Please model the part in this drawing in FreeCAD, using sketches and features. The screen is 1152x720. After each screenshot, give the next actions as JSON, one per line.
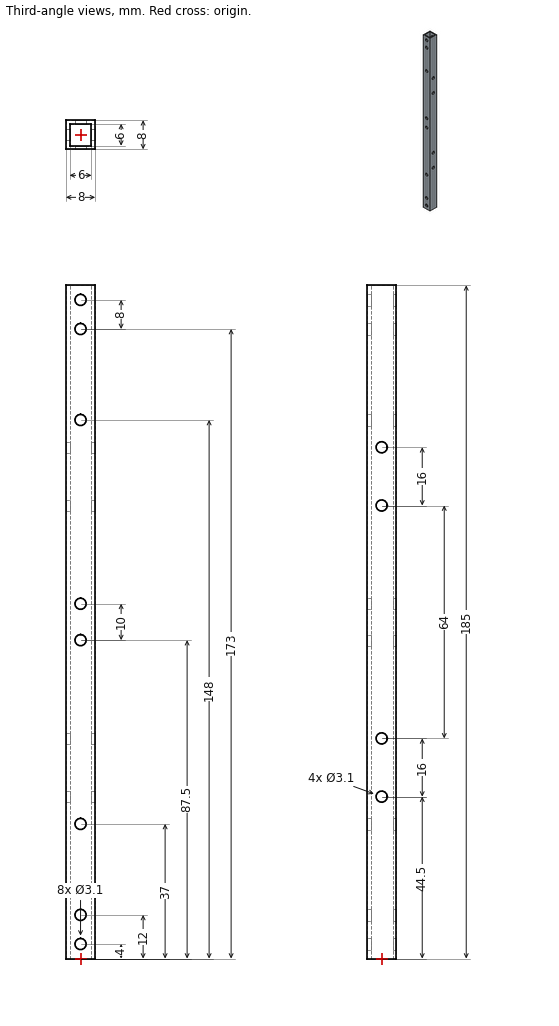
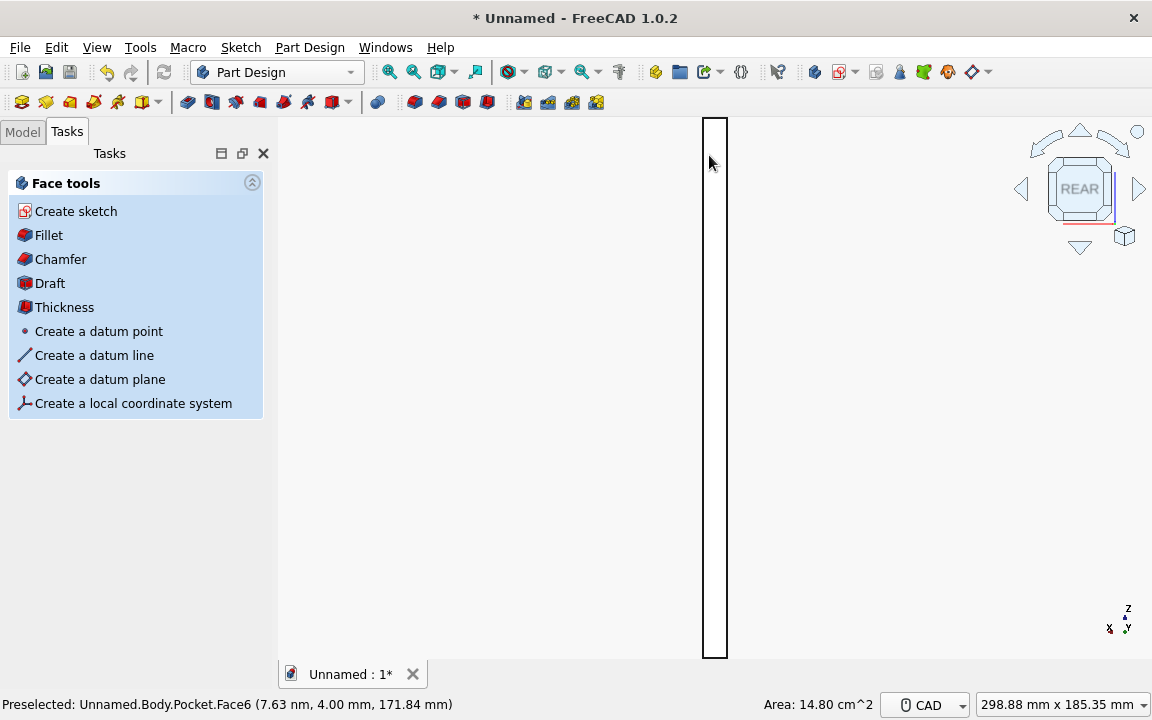
{"action": "left_click", "coordinate": [840, 72]}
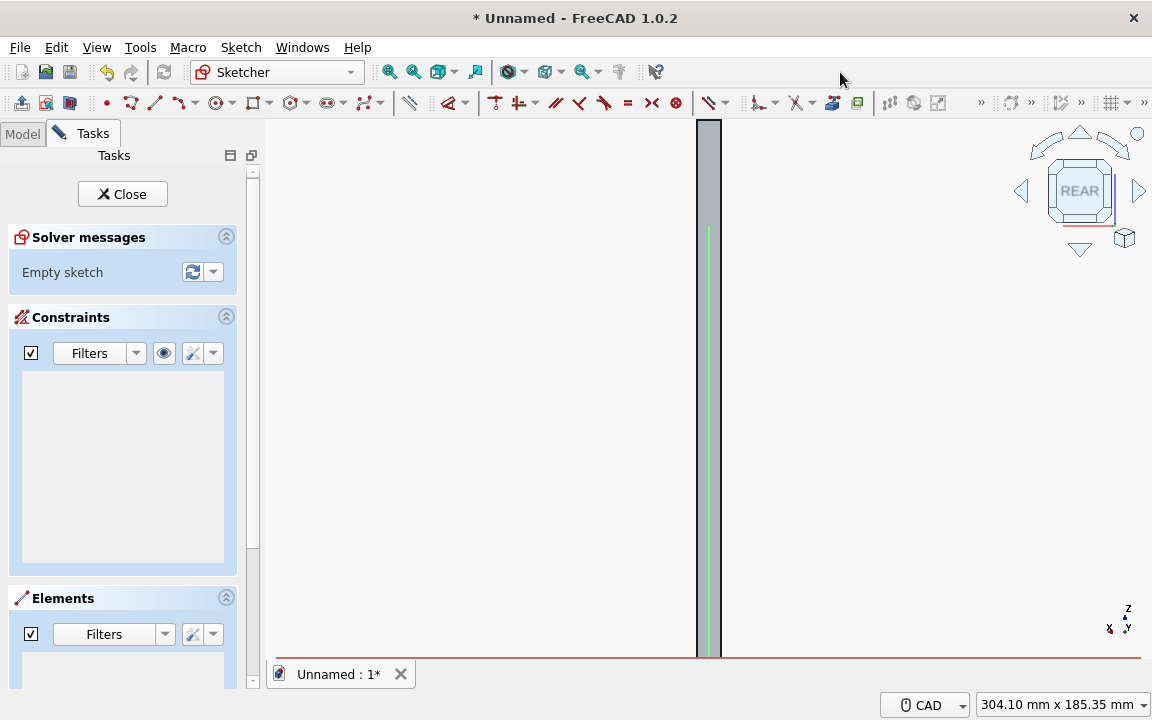
{"action": "scroll", "coordinate": [501, 382], "scroll_direction": "down", "scroll_amount": 2}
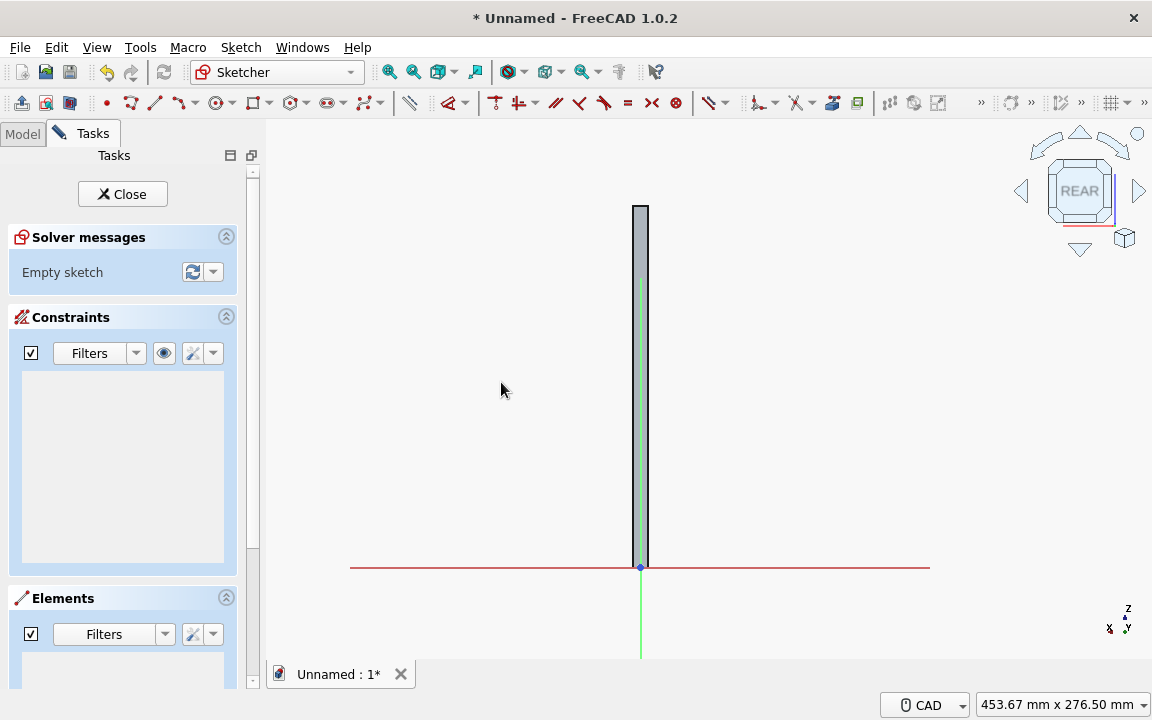
{"action": "left_click", "coordinate": [216, 104]}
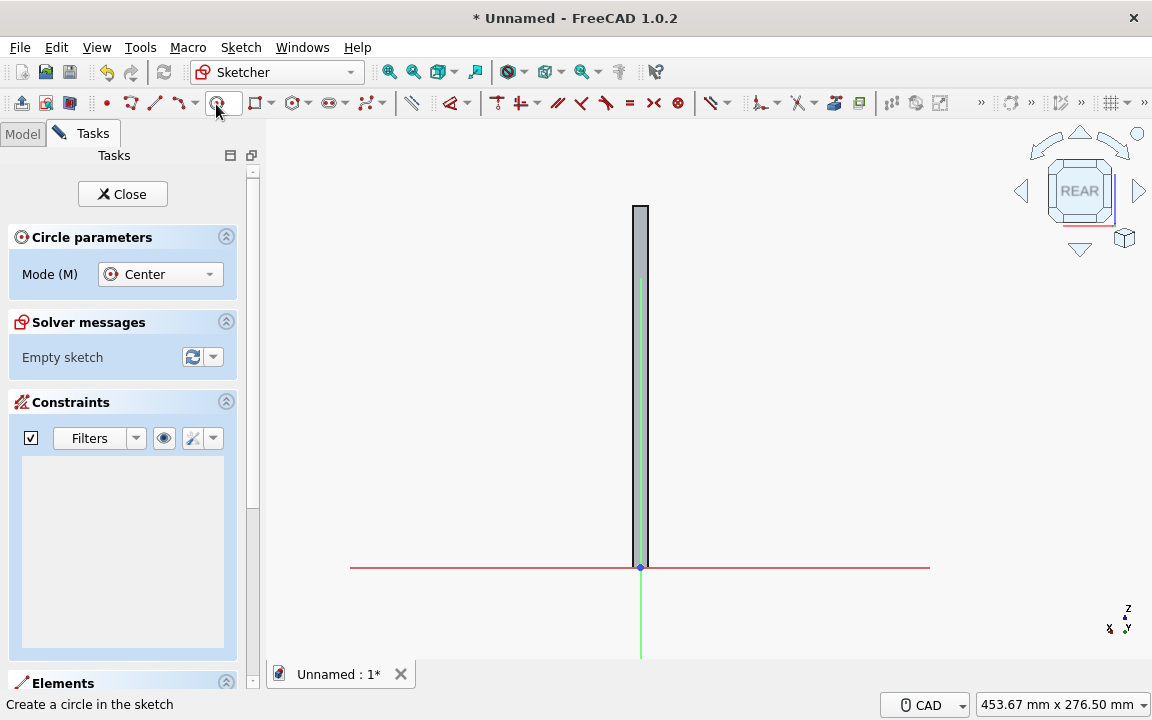
{"action": "scroll", "coordinate": [641, 560], "scroll_direction": "up", "scroll_amount": 11}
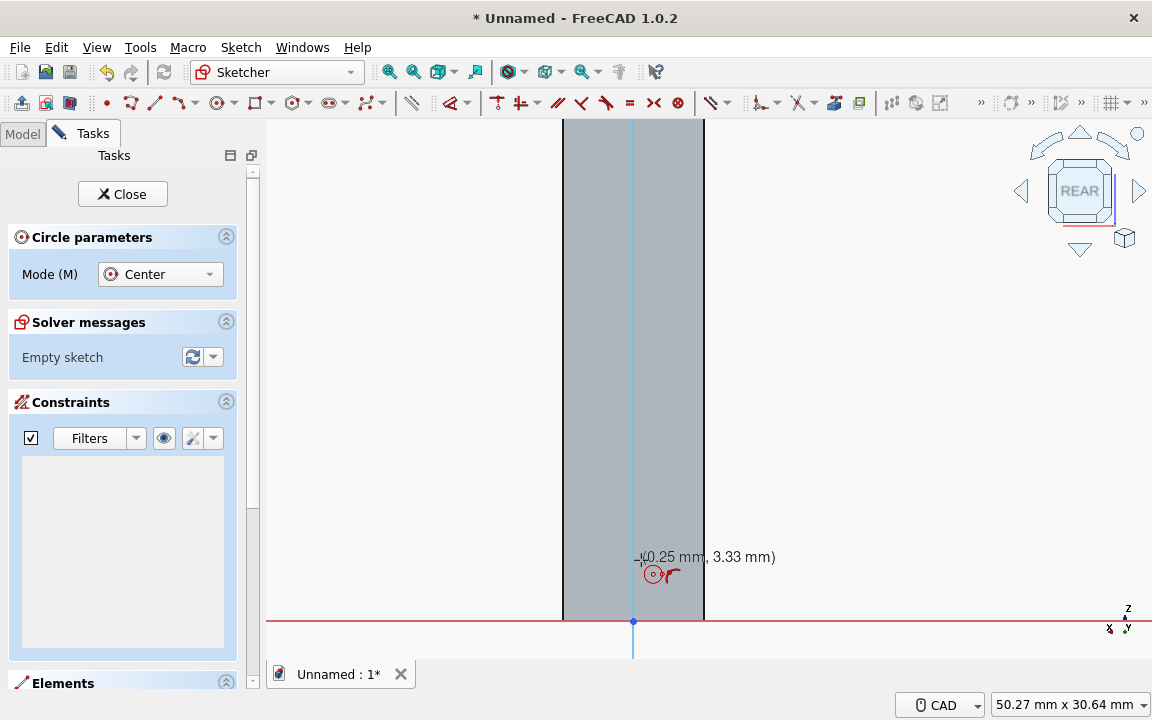
{"action": "scroll", "coordinate": [641, 561], "scroll_direction": "down", "scroll_amount": 11}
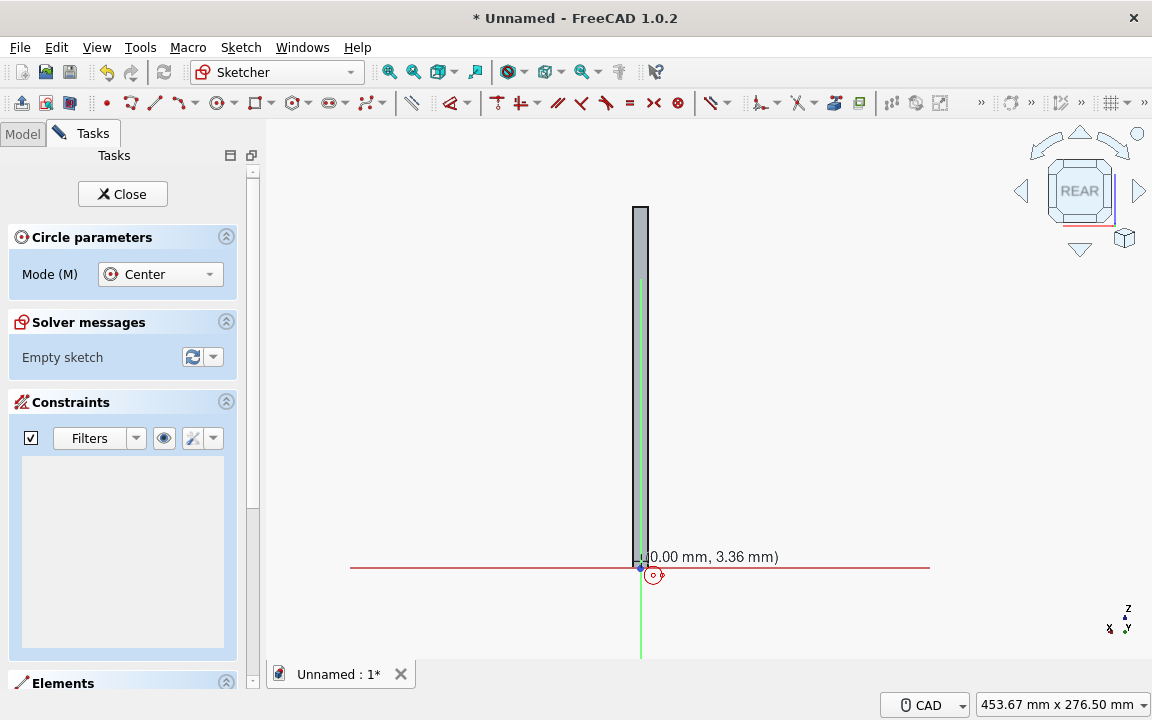
{"action": "scroll", "coordinate": [641, 561], "scroll_direction": "up", "scroll_amount": 4}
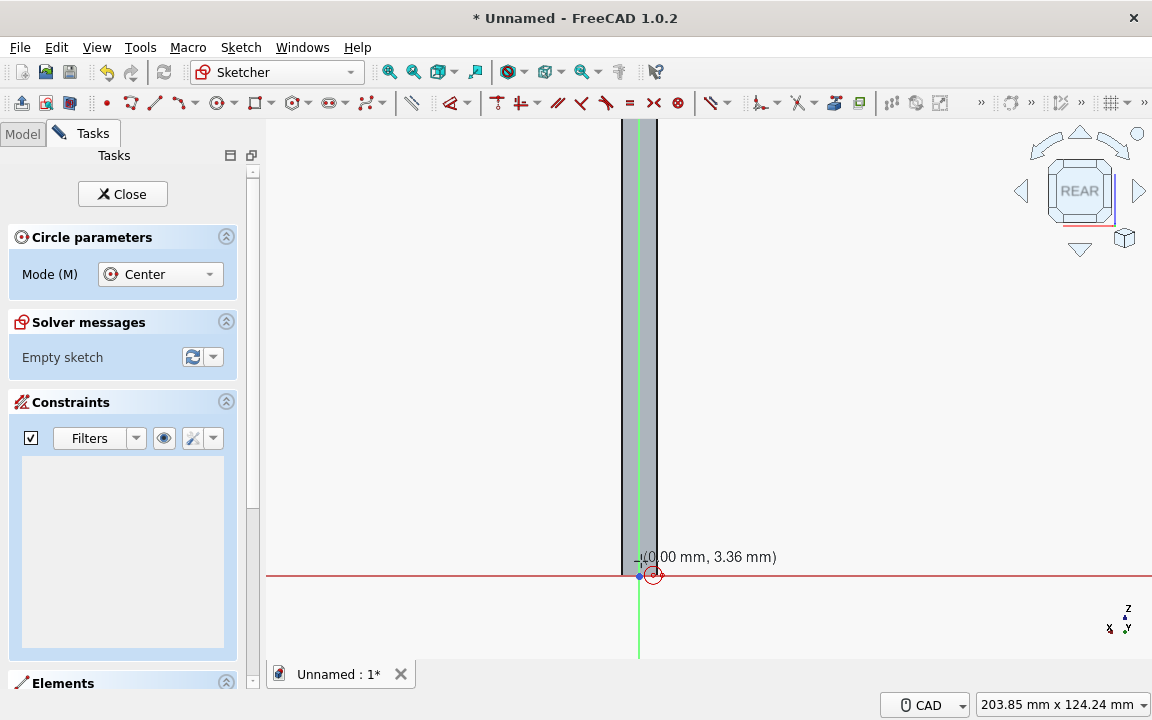
{"action": "left_click", "coordinate": [639, 559]}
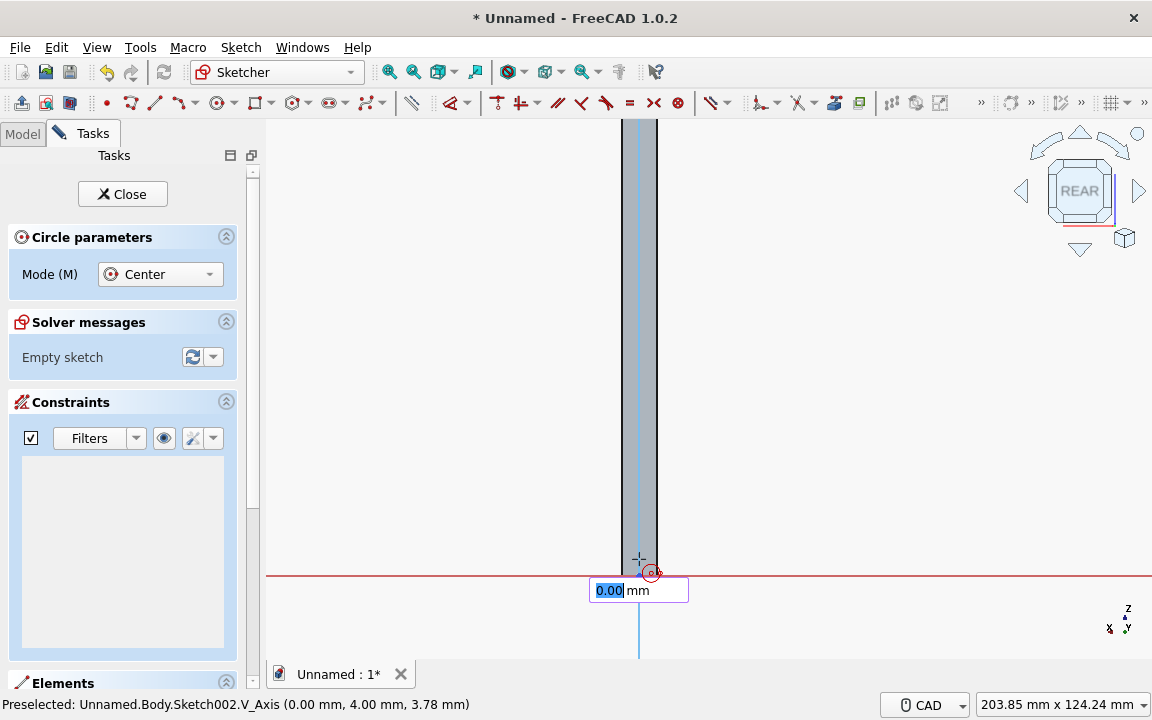
{"action": "scroll", "coordinate": [646, 557], "scroll_direction": "up", "scroll_amount": 5}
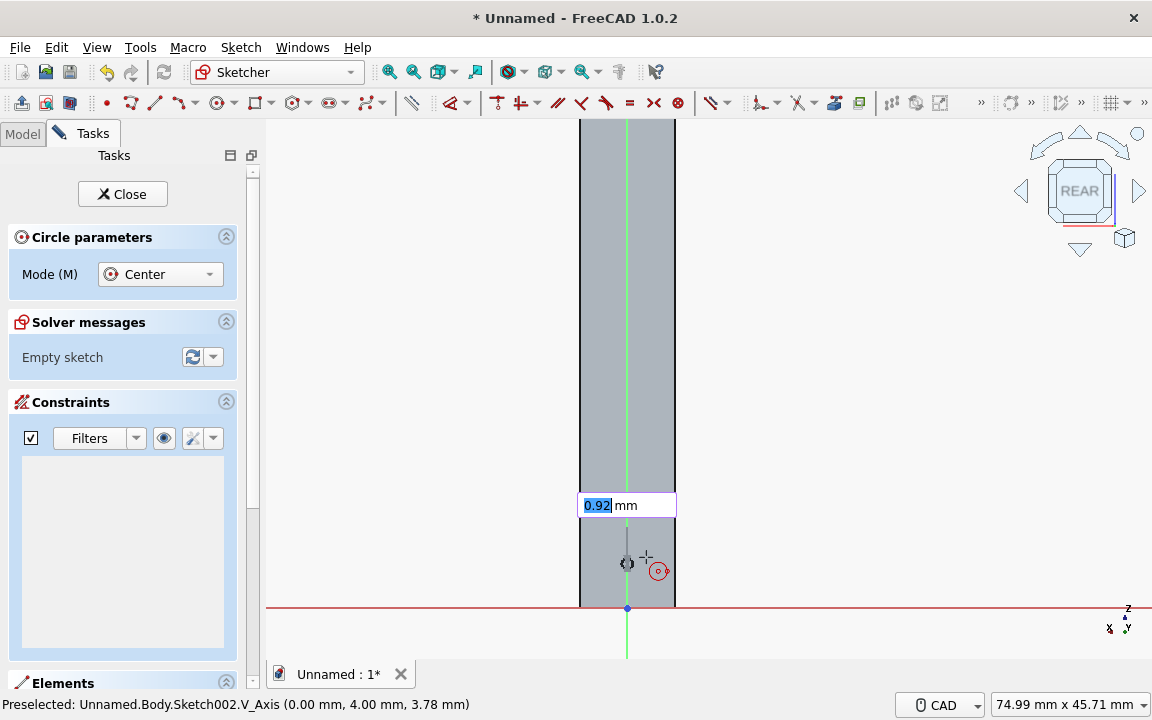
{"action": "left_click", "coordinate": [645, 555]}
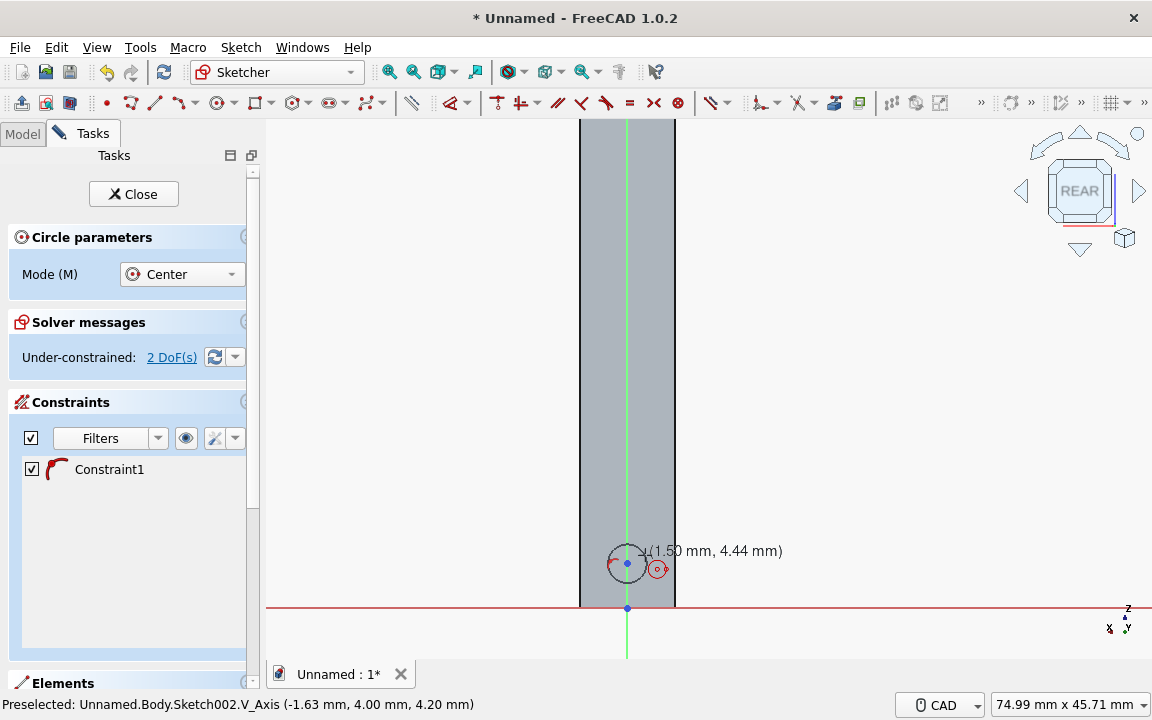
{"action": "scroll", "coordinate": [627, 467], "scroll_direction": "up", "scroll_amount": 2}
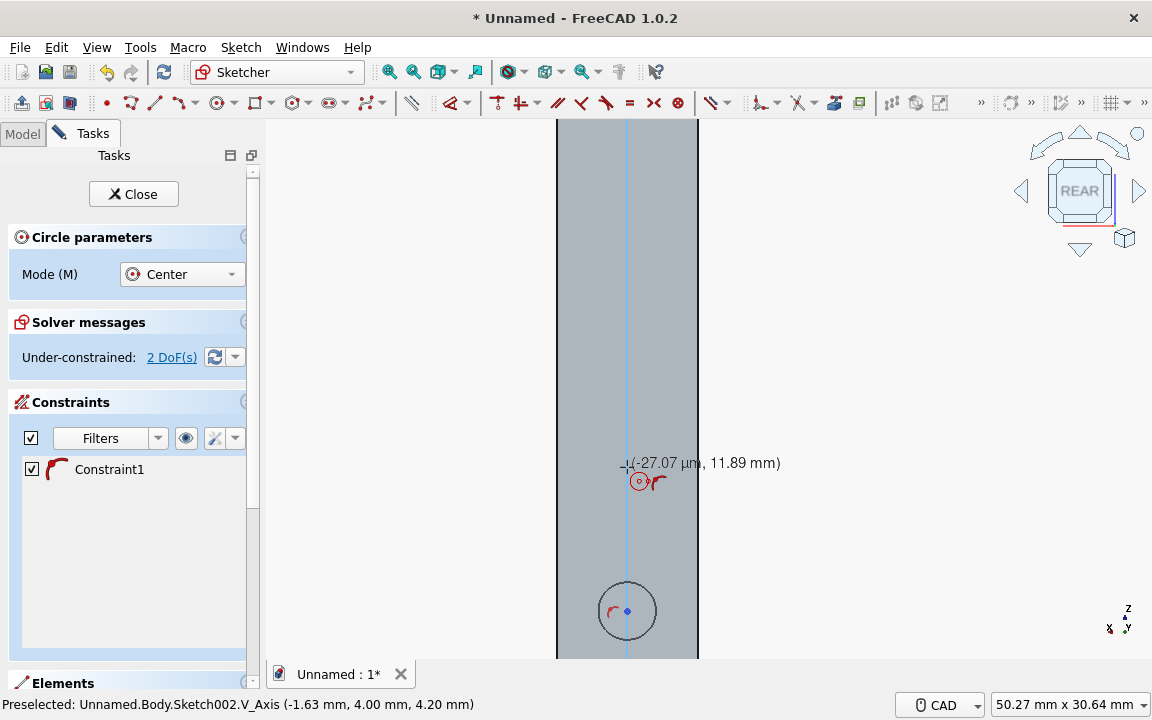
{"action": "scroll", "coordinate": [642, 553], "scroll_direction": "down", "scroll_amount": 11}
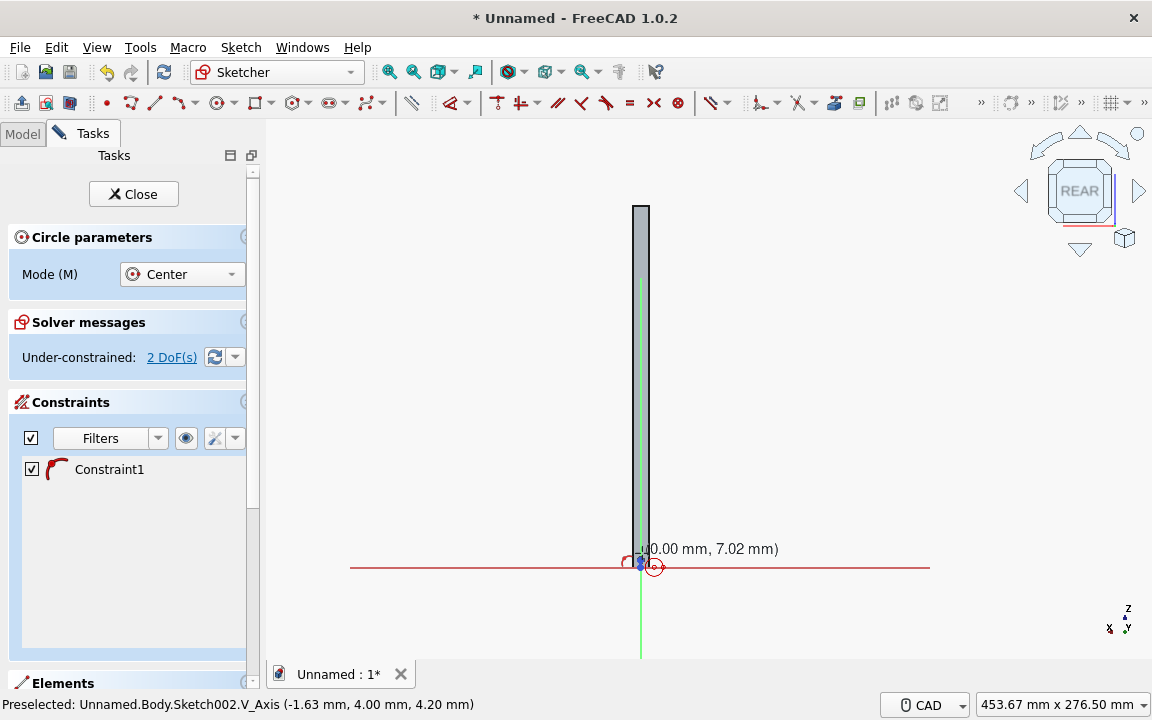
{"action": "scroll", "coordinate": [641, 544], "scroll_direction": "up", "scroll_amount": 2}